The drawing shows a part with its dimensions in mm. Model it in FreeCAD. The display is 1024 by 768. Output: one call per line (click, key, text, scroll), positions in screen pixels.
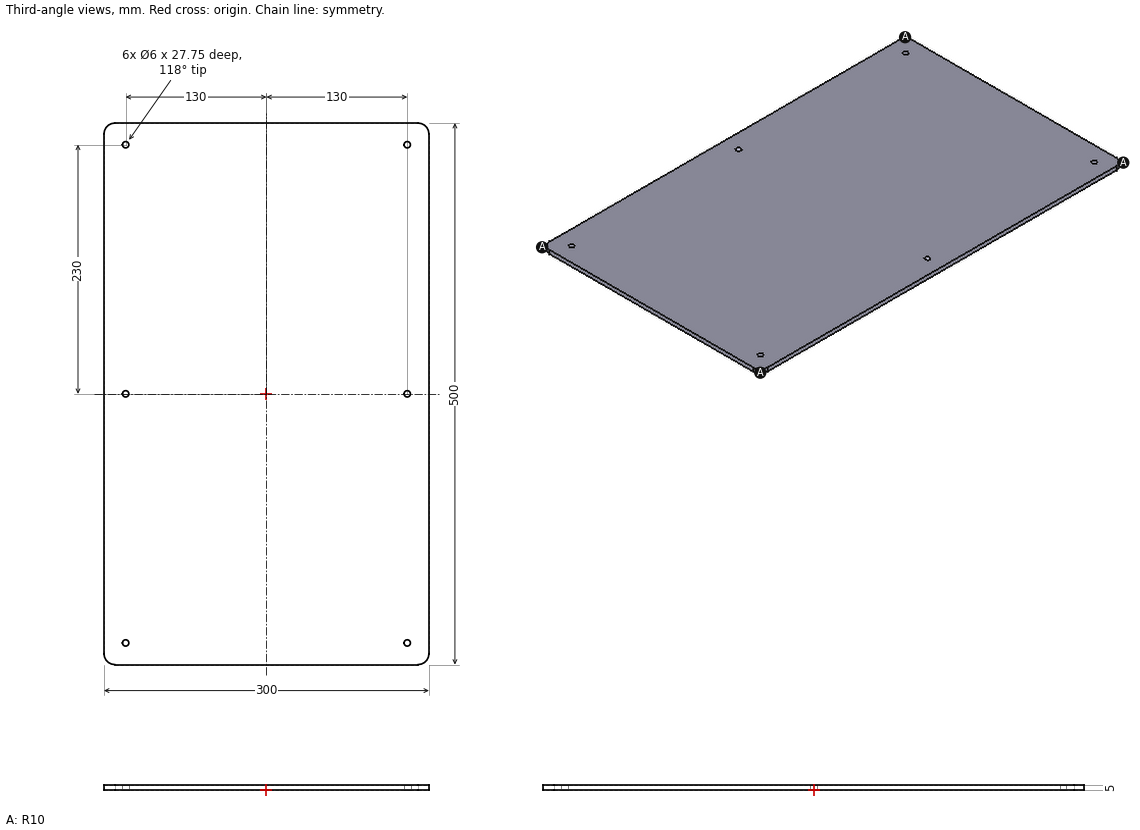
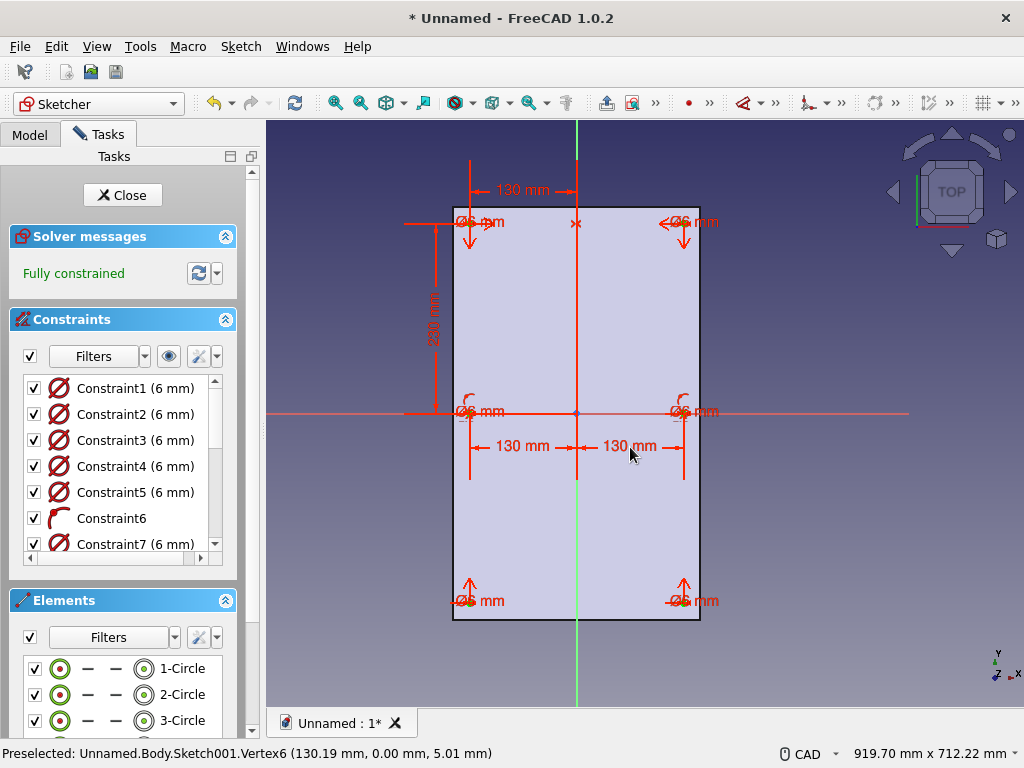
click(123, 195)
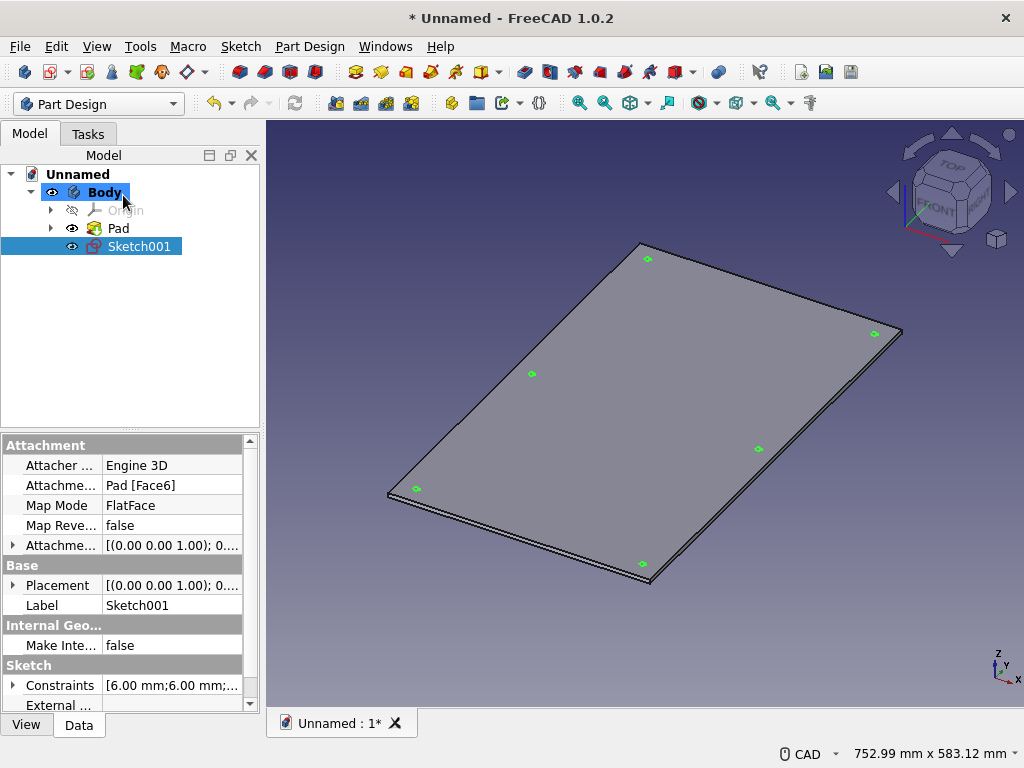
click(550, 72)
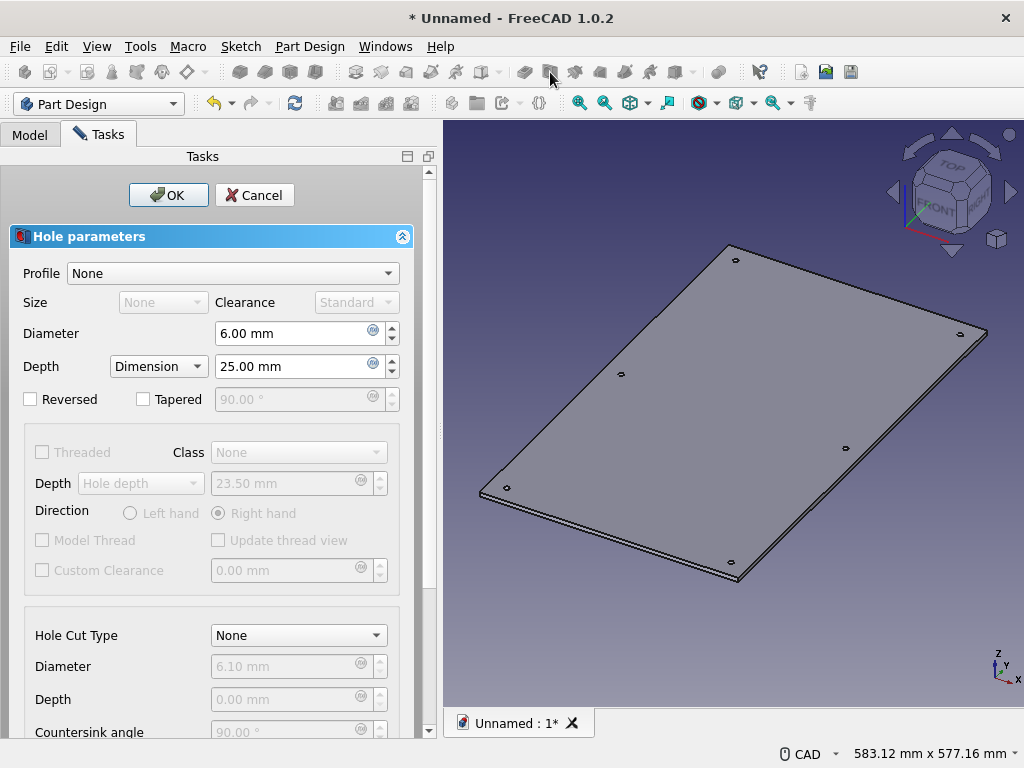
triple_click(300, 334)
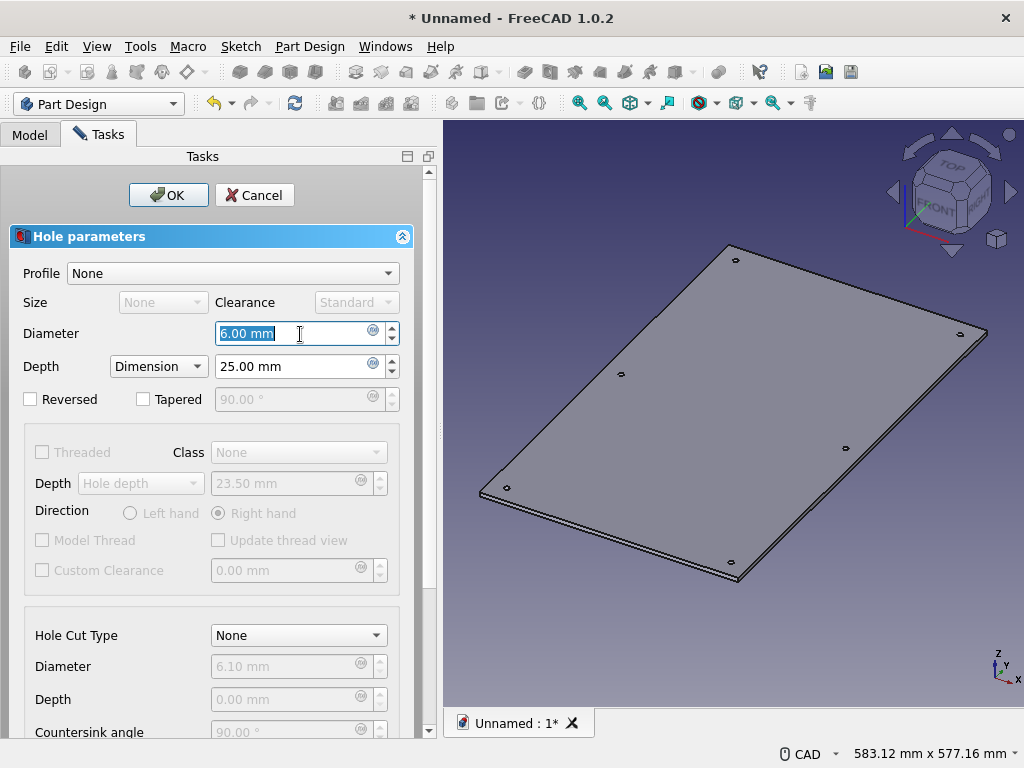
text(6)
key(Tab)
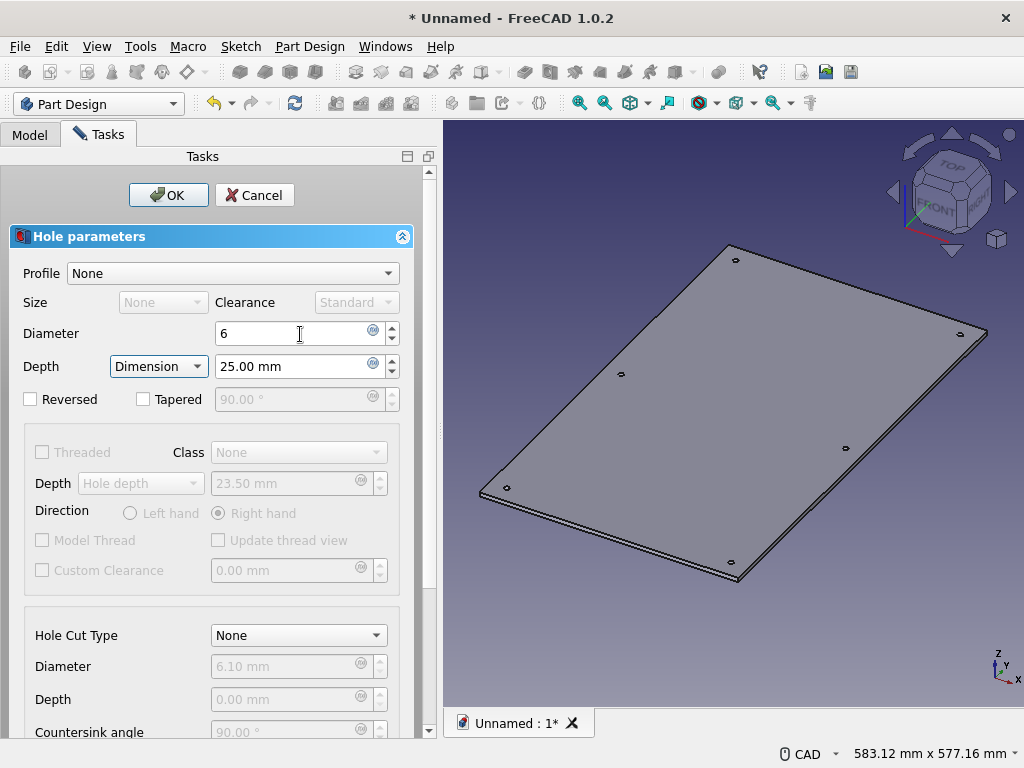
triple_click(300, 366)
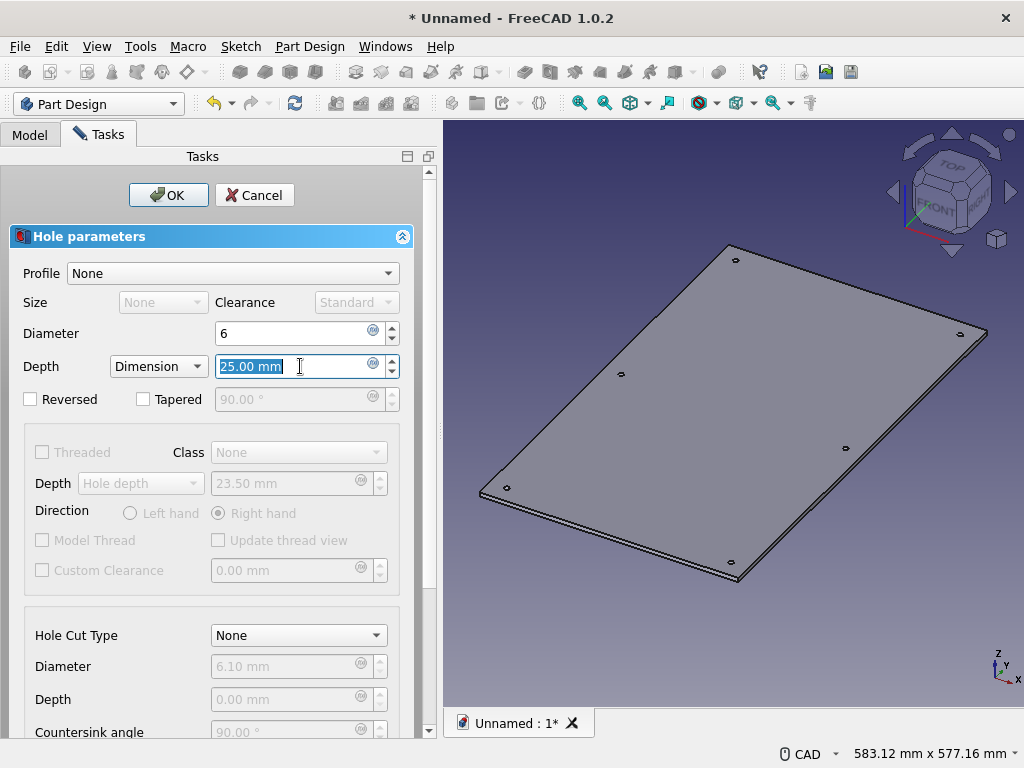
text(27.75)
key(Tab)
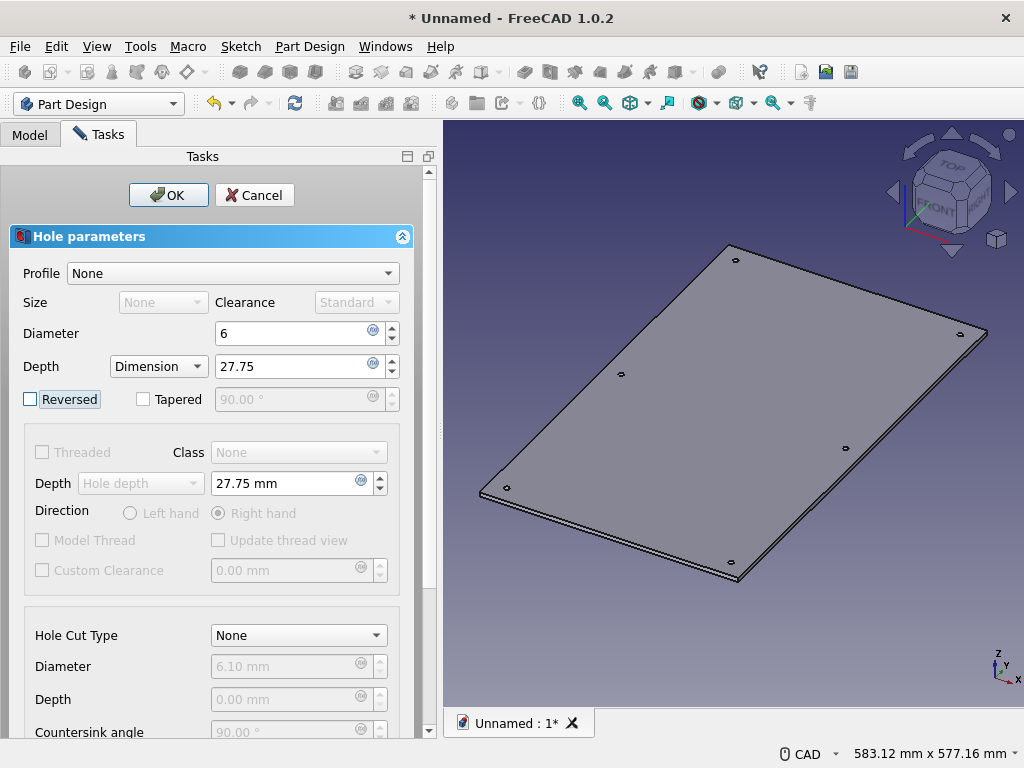
click(169, 195)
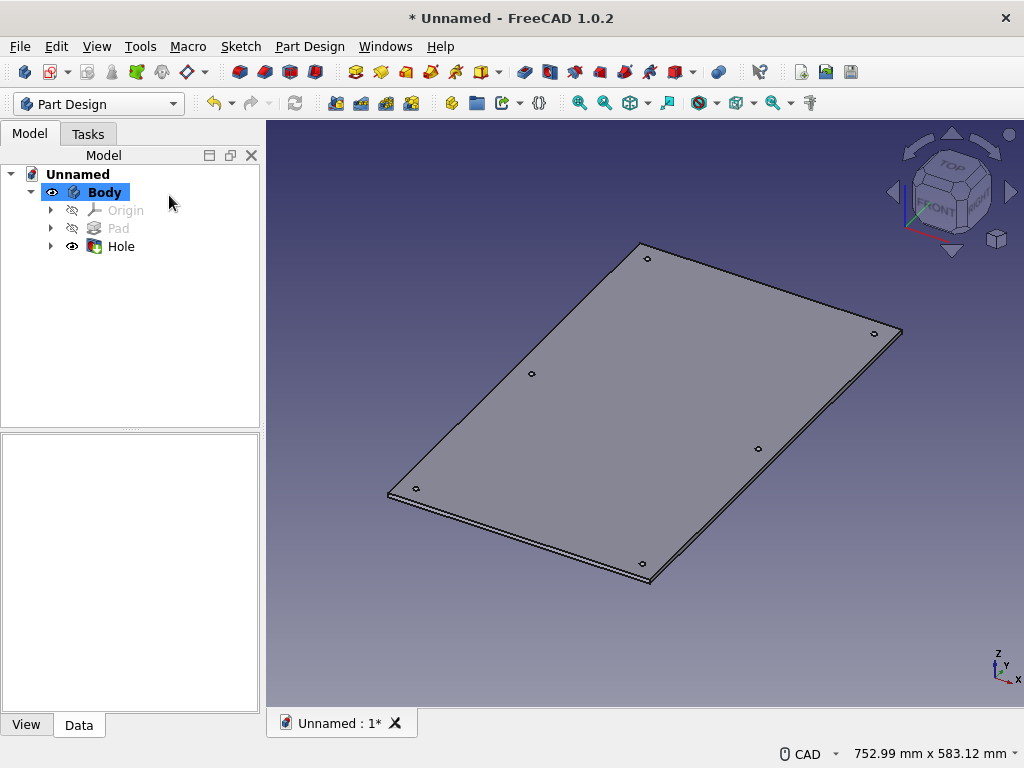
scroll(650, 581, up, 11)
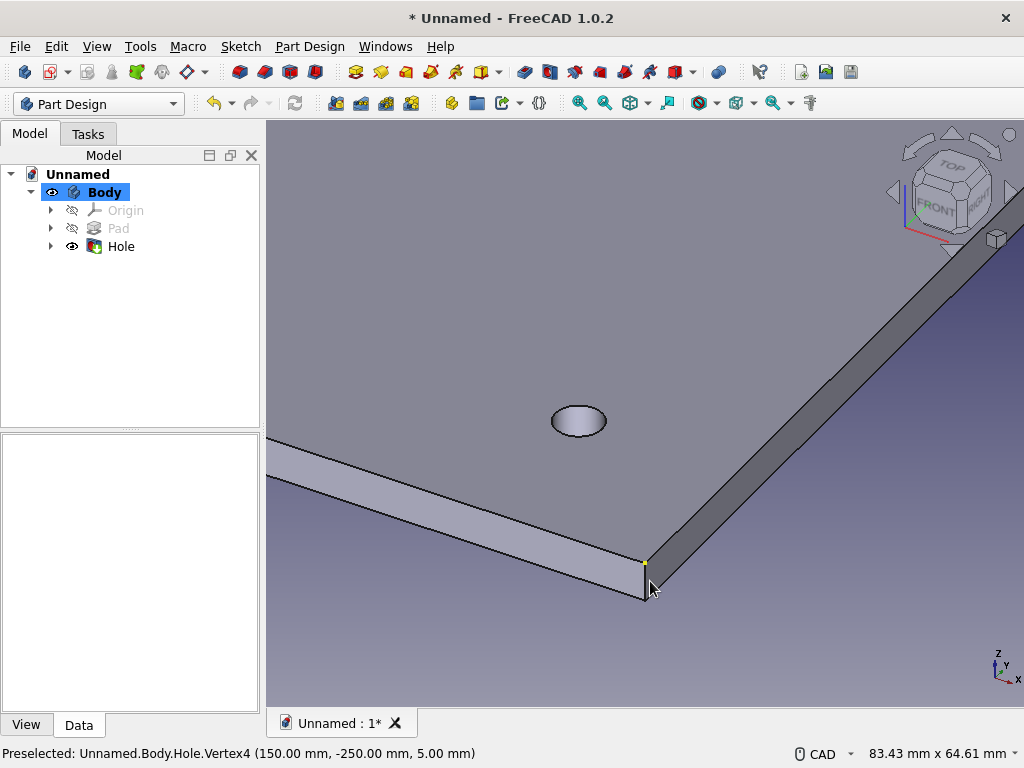
click(645, 581)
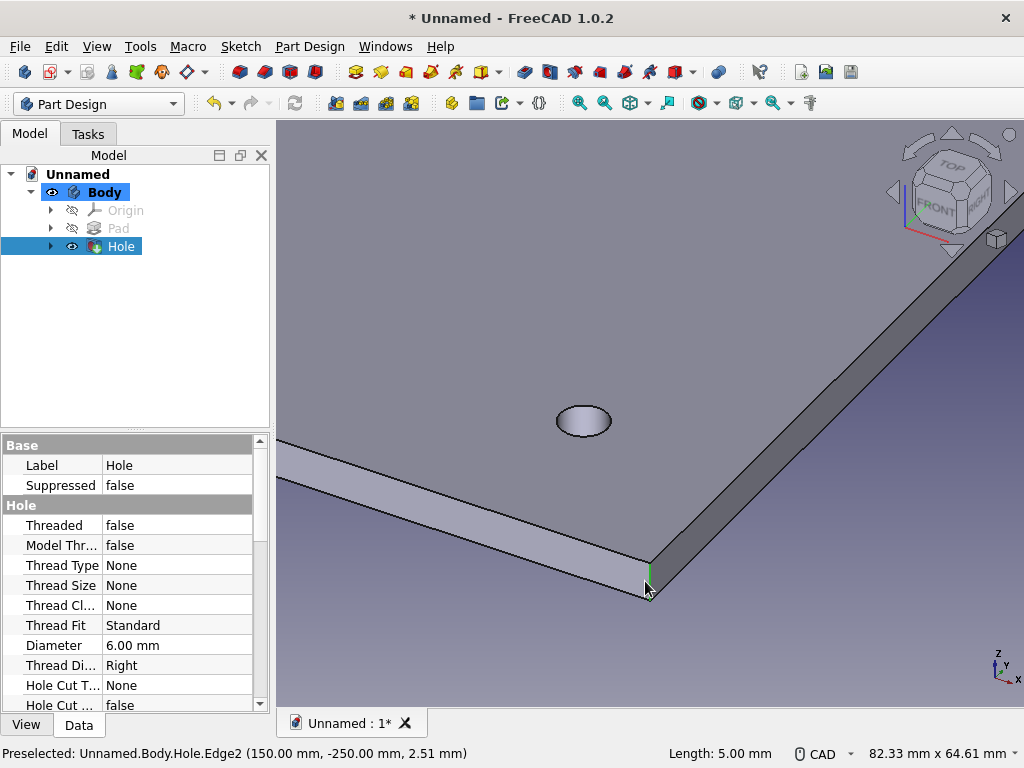
click(580, 104)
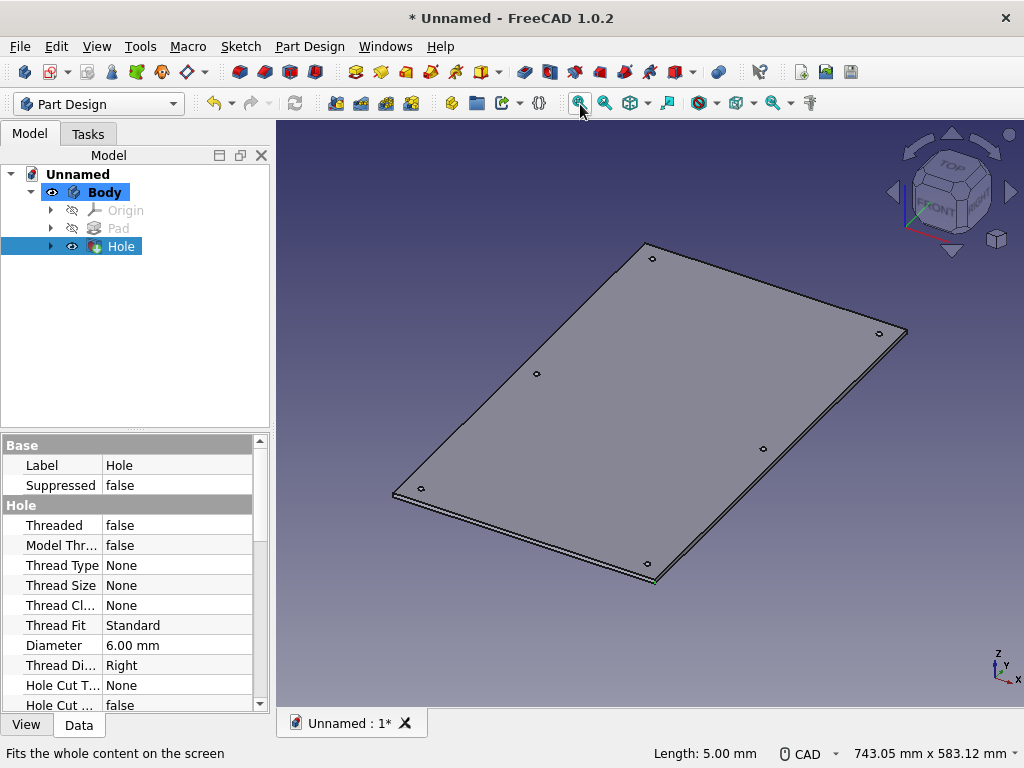
key(0)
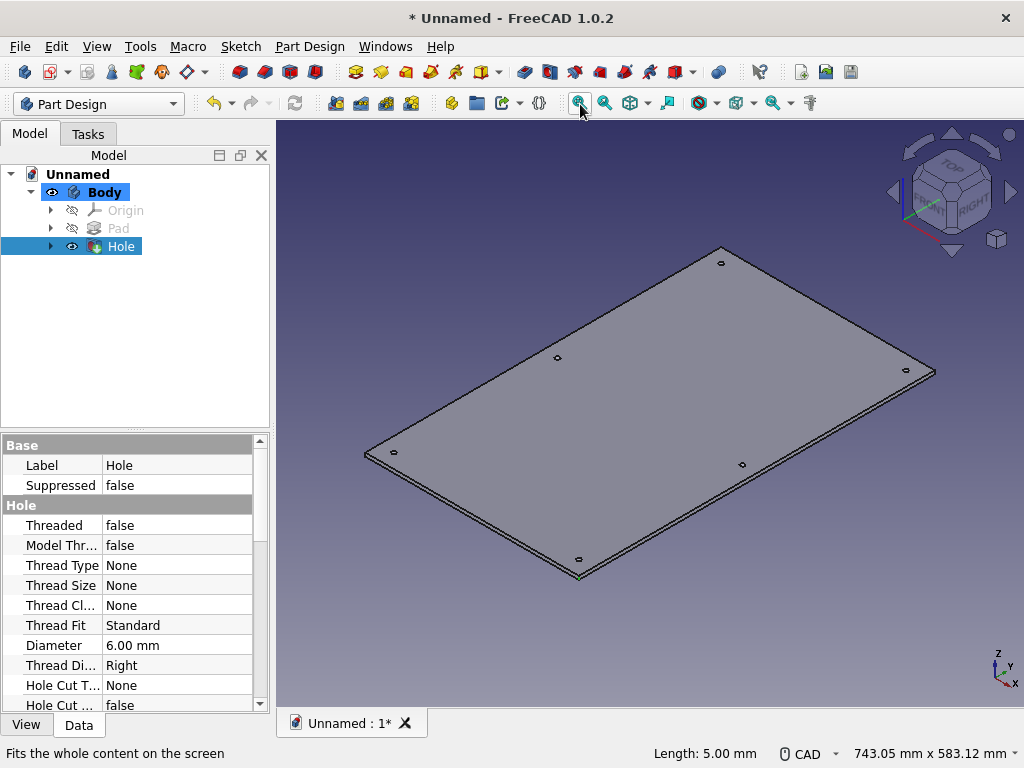
scroll(365, 454, up, 11)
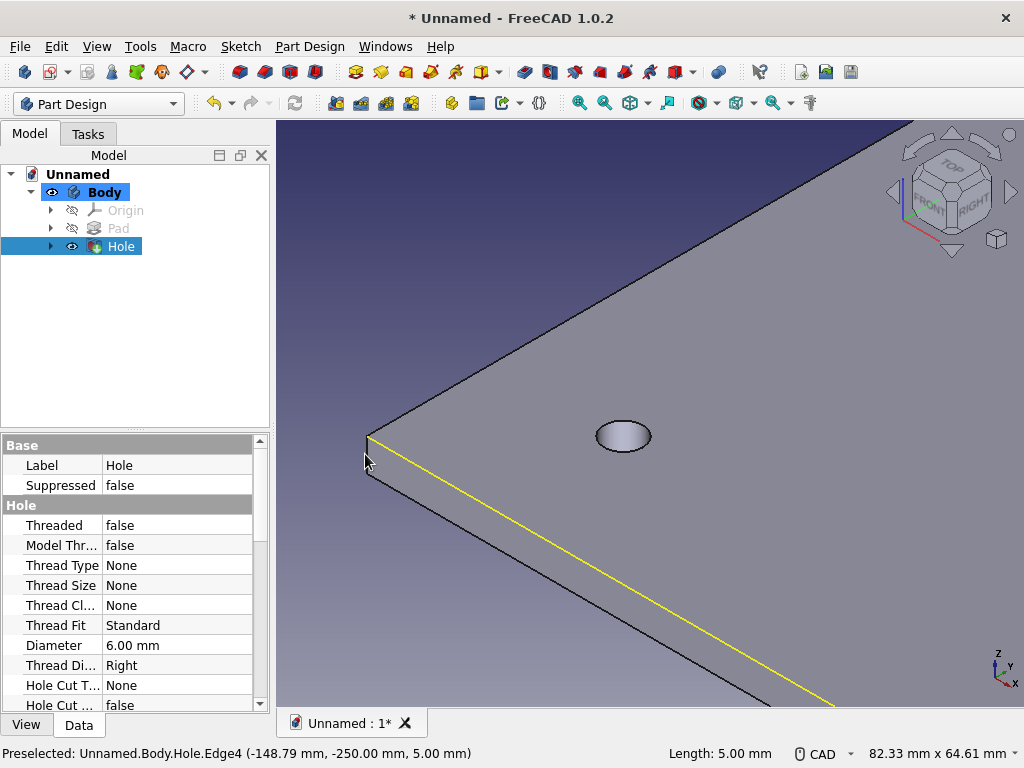
click(580, 104)